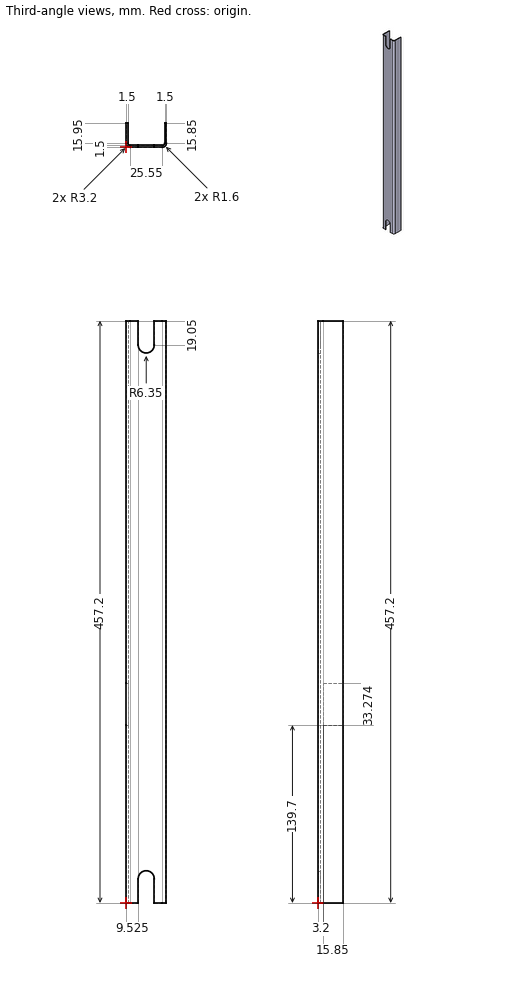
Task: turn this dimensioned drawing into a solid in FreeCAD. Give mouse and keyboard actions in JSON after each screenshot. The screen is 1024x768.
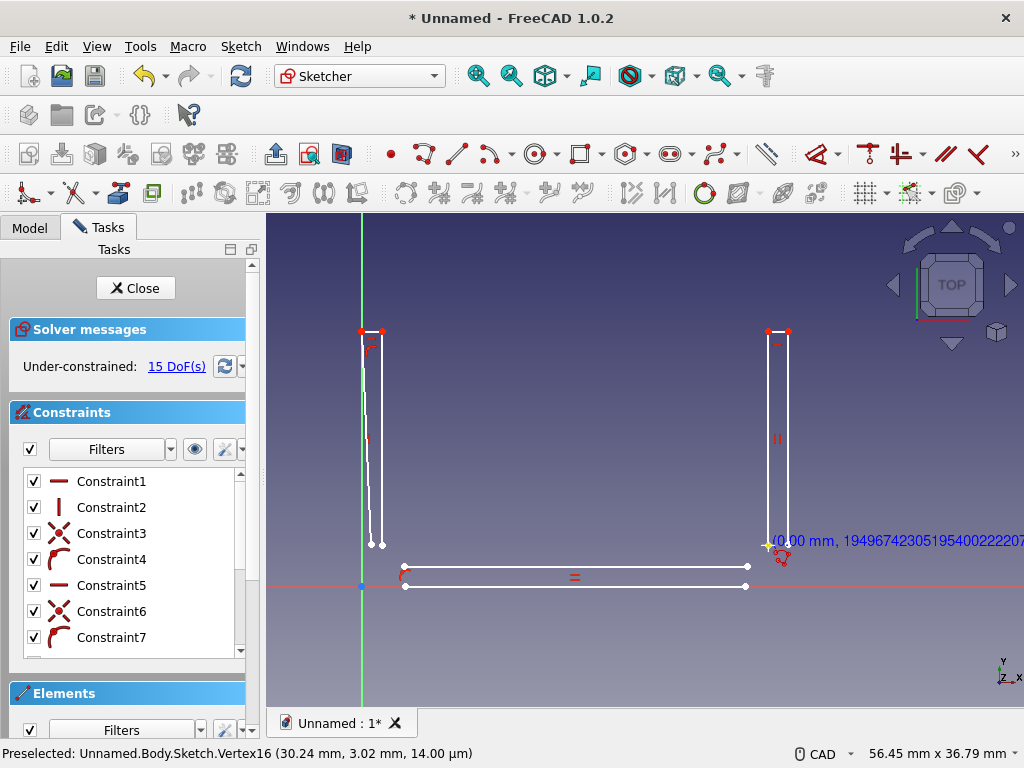
{"action": "key", "text": "g 3 a"}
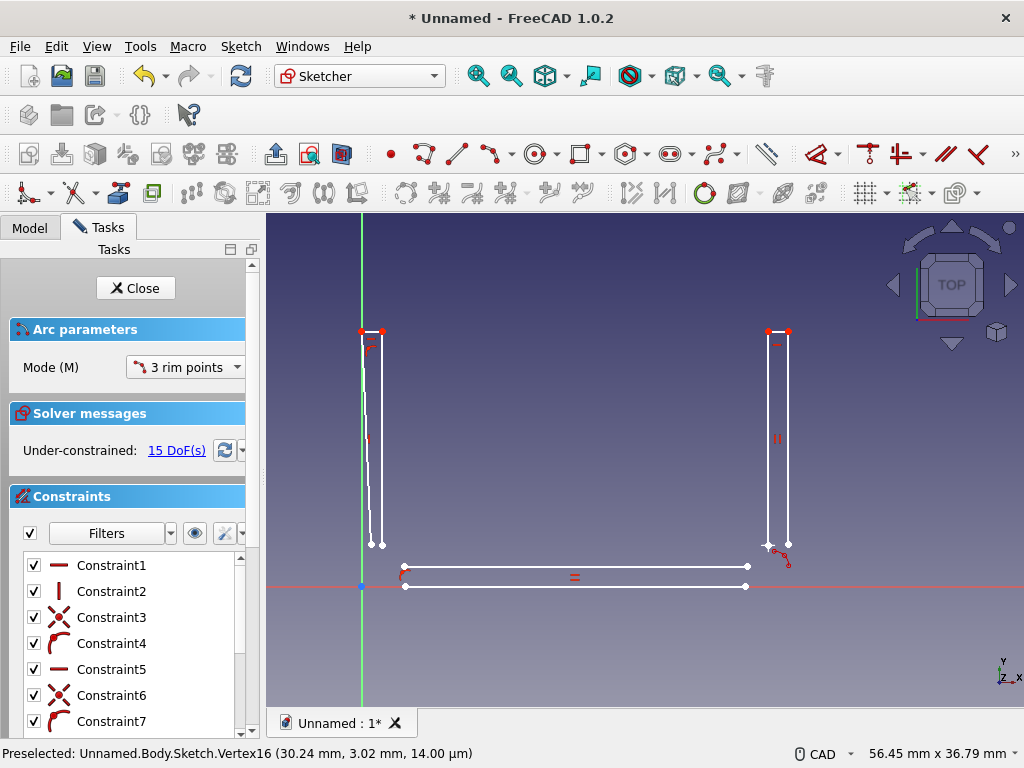
{"action": "left_click", "coordinate": [404, 567]}
{"action": "left_click", "coordinate": [382, 546]}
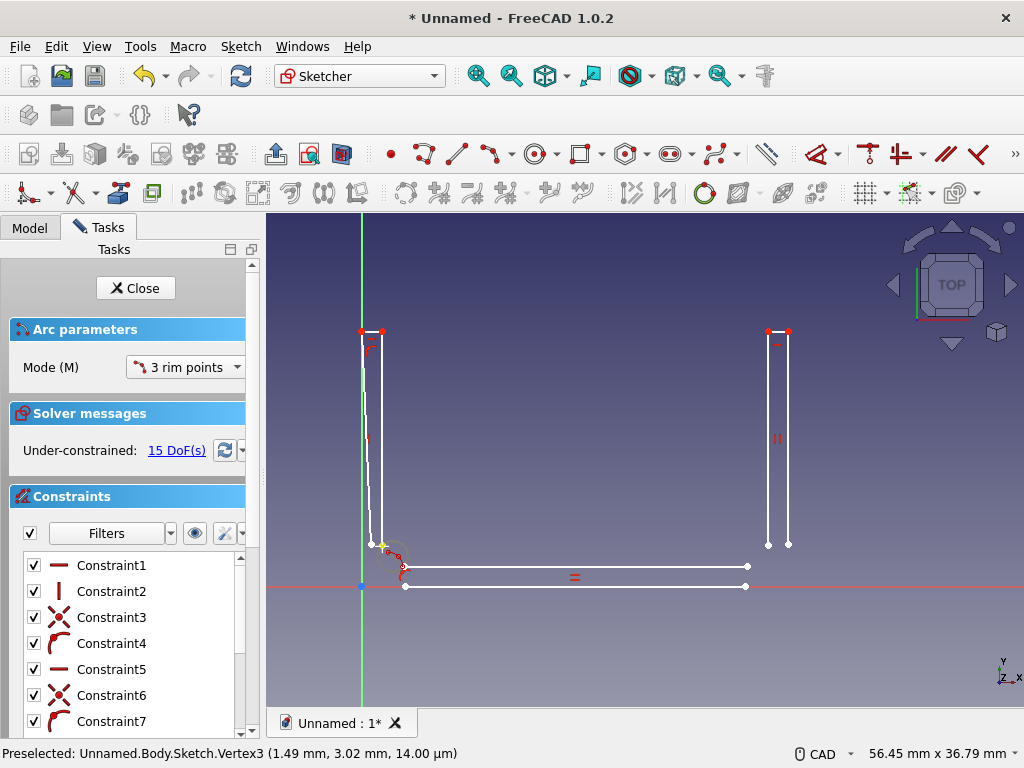
{"action": "scroll", "coordinate": [388, 560], "scroll_direction": "up", "scroll_amount": 5}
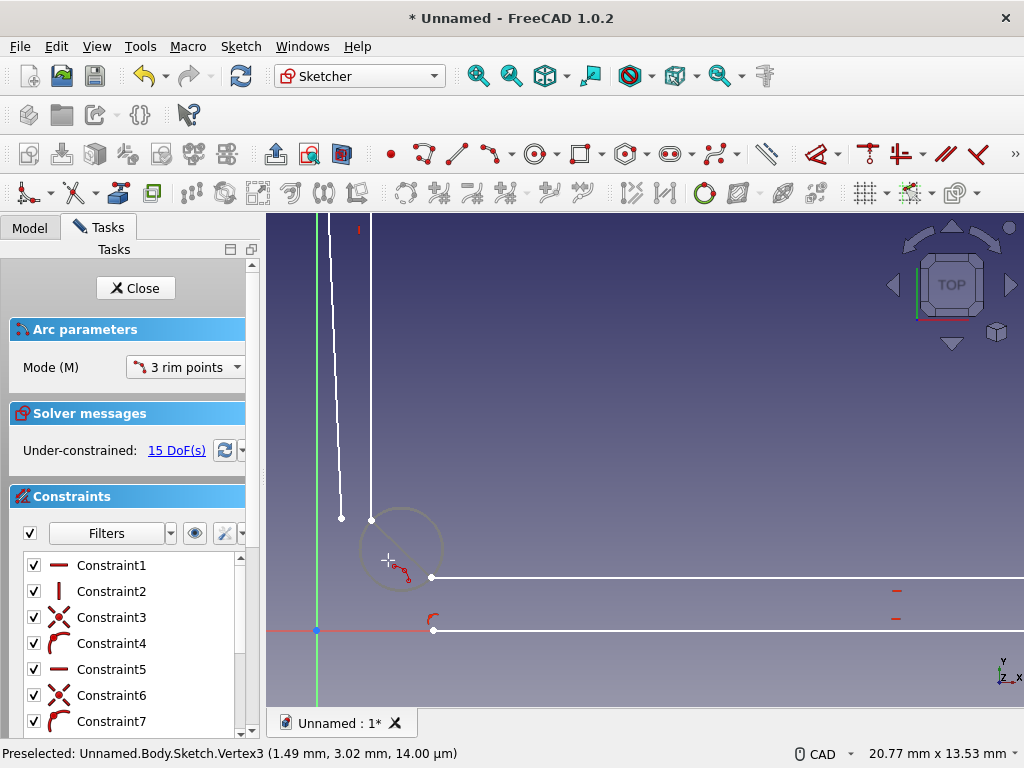
{"action": "left_click", "coordinate": [389, 559]}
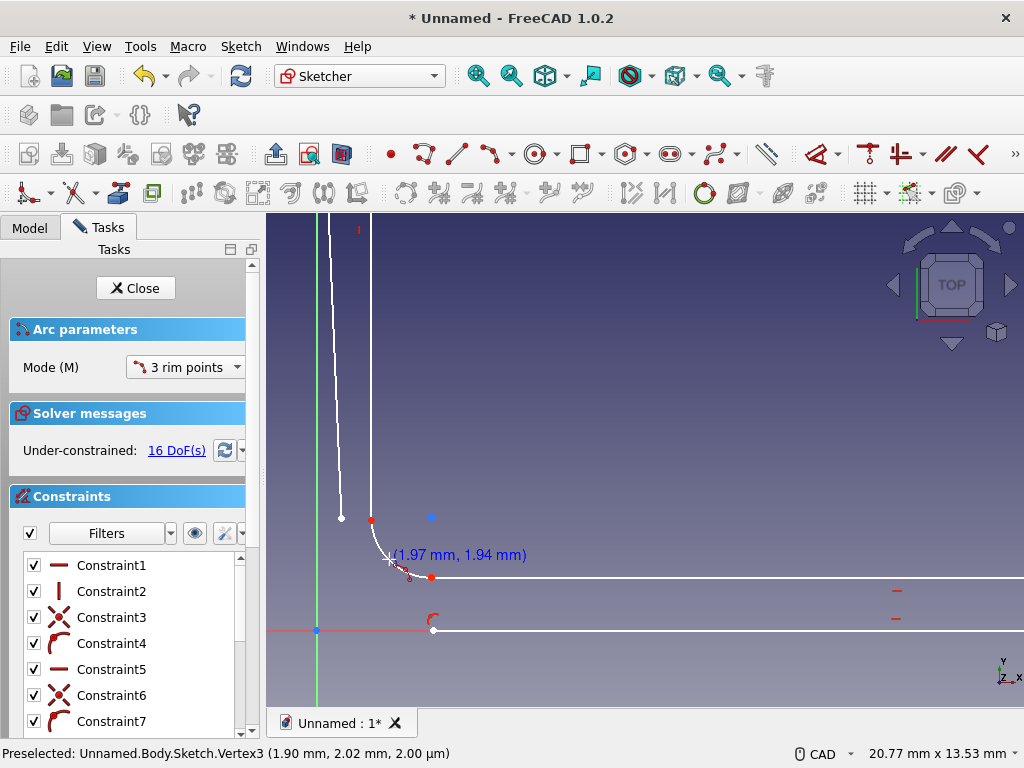
{"action": "left_click", "coordinate": [342, 518]}
{"action": "left_click", "coordinate": [434, 631]}
{"action": "left_click", "coordinate": [351, 597]}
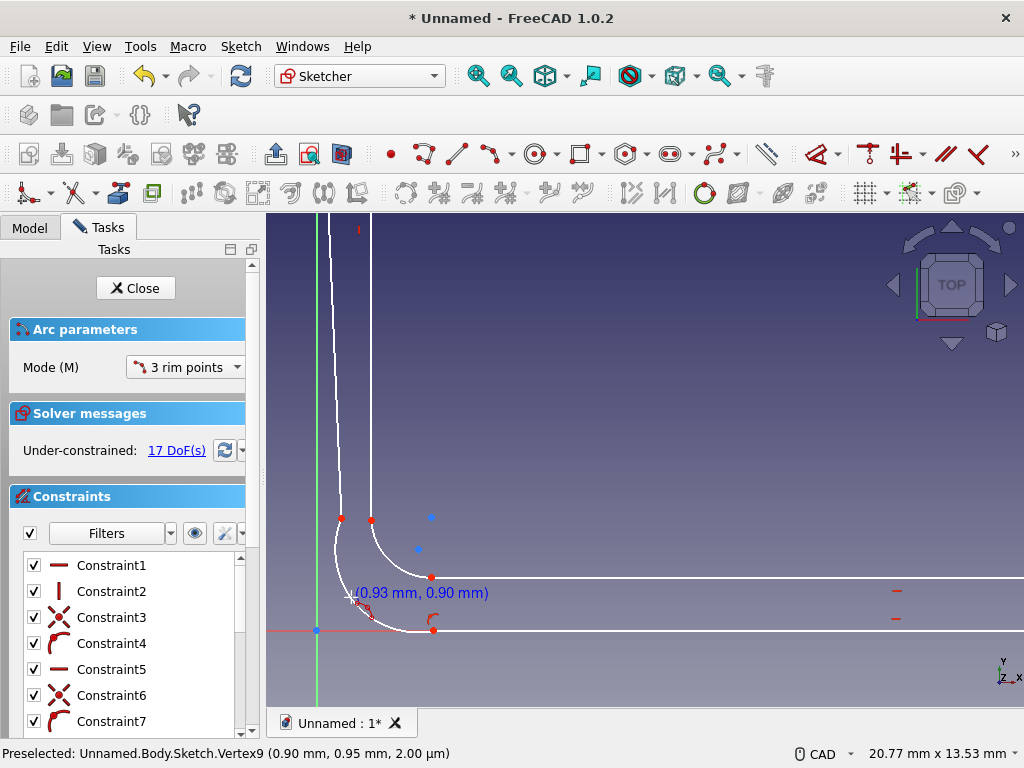
{"action": "scroll", "coordinate": [390, 563], "scroll_direction": "down", "scroll_amount": 5}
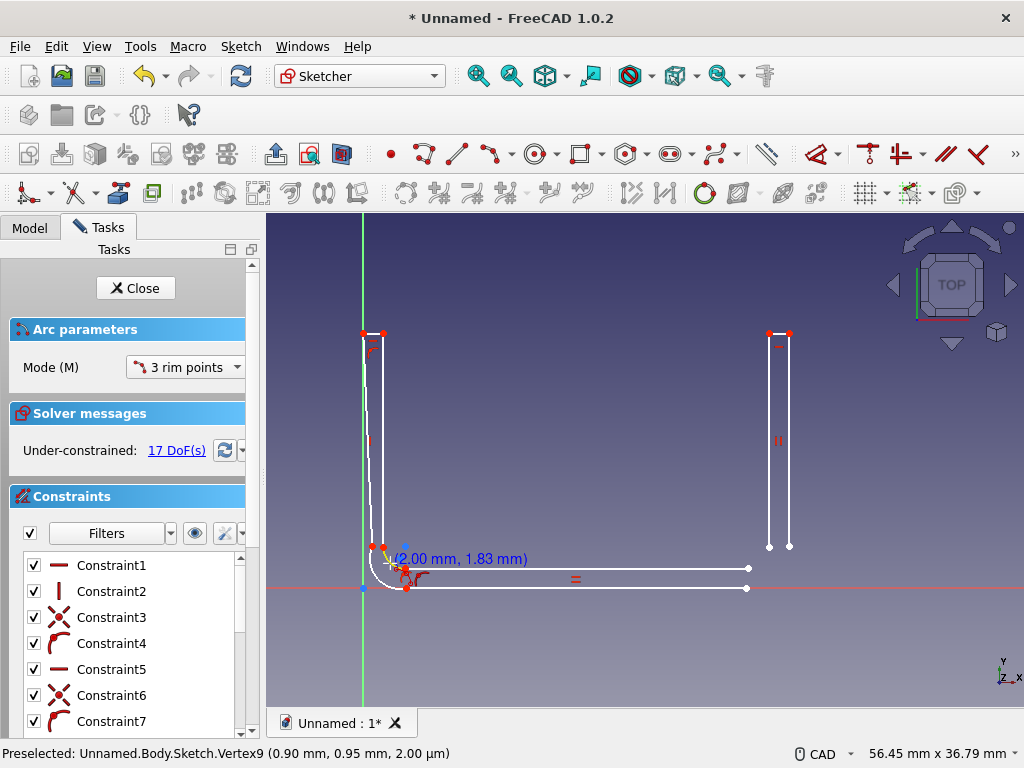
{"action": "left_click", "coordinate": [746, 588]}
{"action": "left_click", "coordinate": [789, 547]}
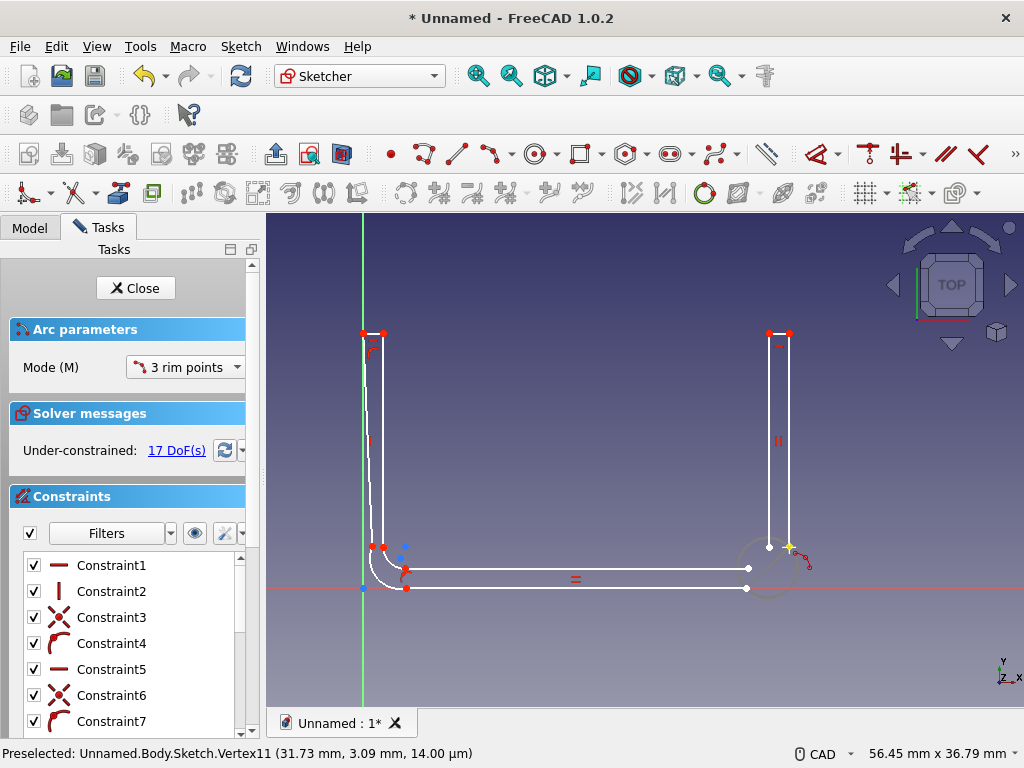
{"action": "scroll", "coordinate": [777, 576], "scroll_direction": "up", "scroll_amount": 2}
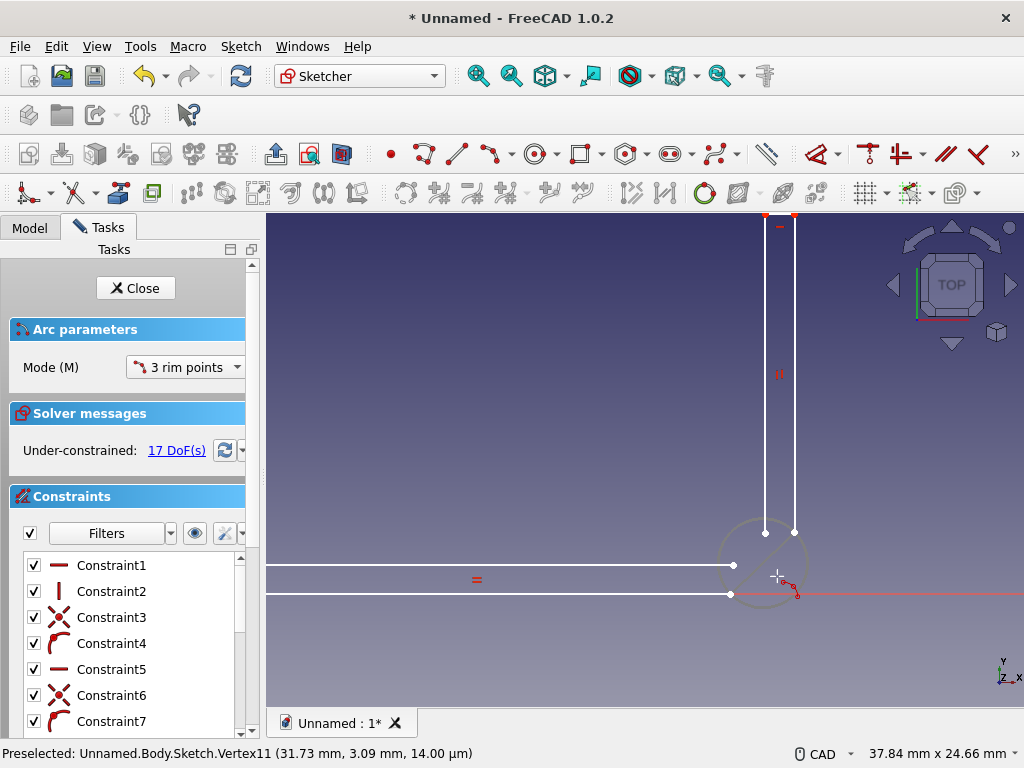
{"action": "left_click", "coordinate": [777, 575]}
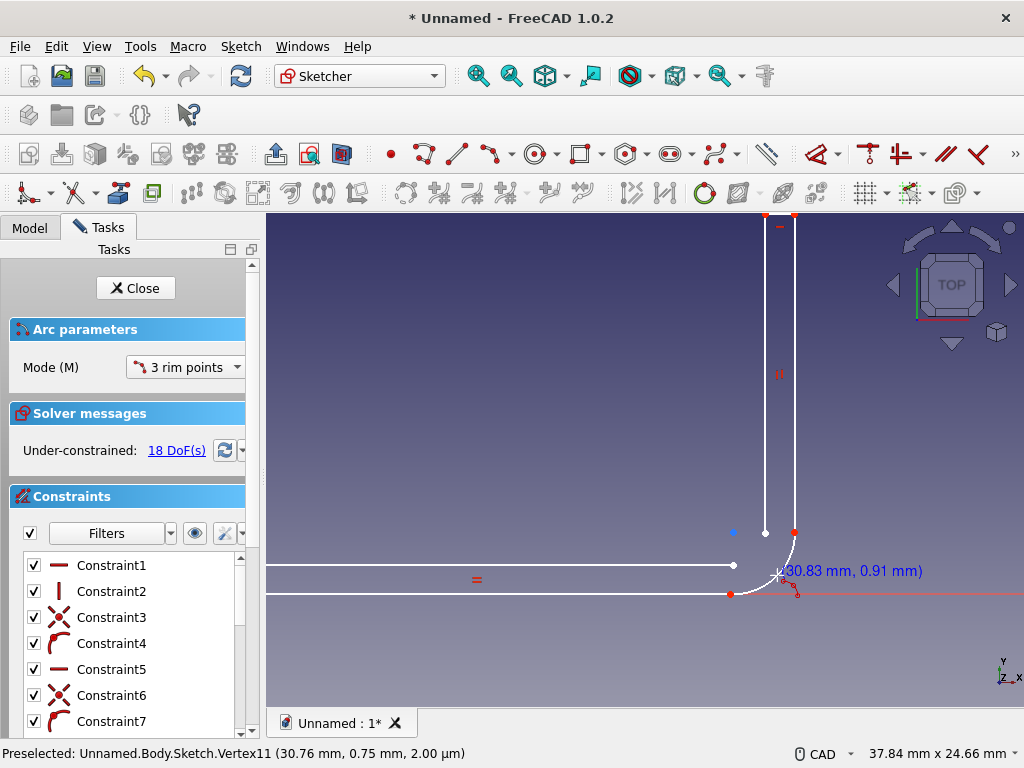
{"action": "left_click", "coordinate": [765, 534]}
{"action": "left_click", "coordinate": [734, 565]}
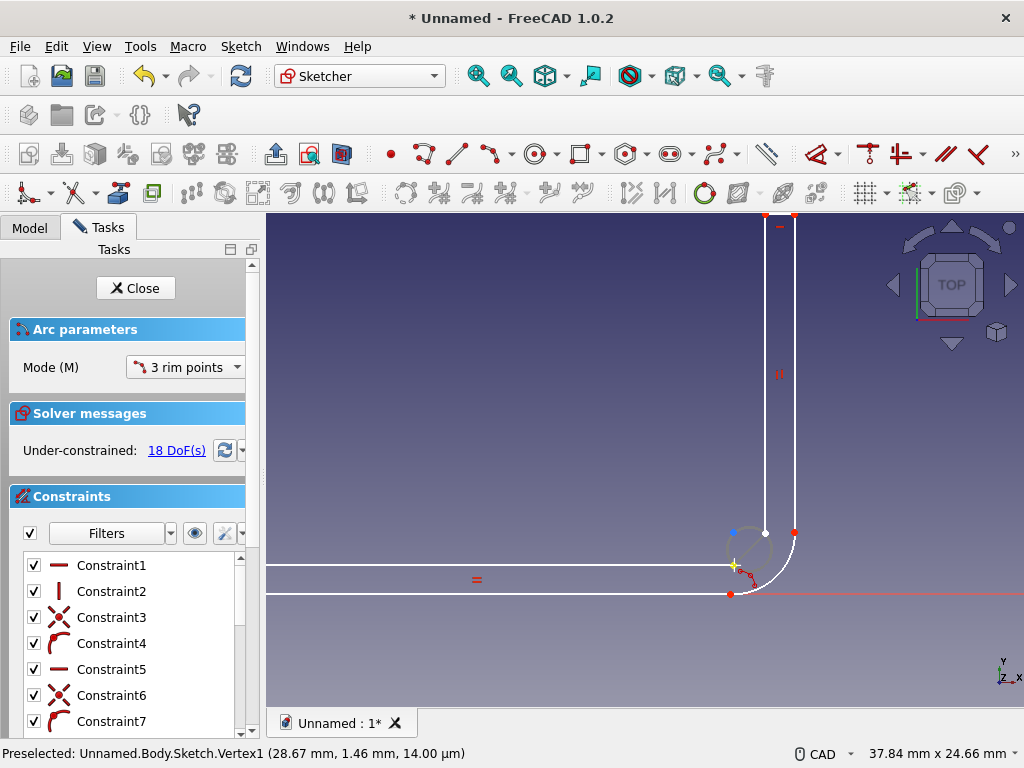
{"action": "scroll", "coordinate": [756, 555], "scroll_direction": "up", "scroll_amount": 3}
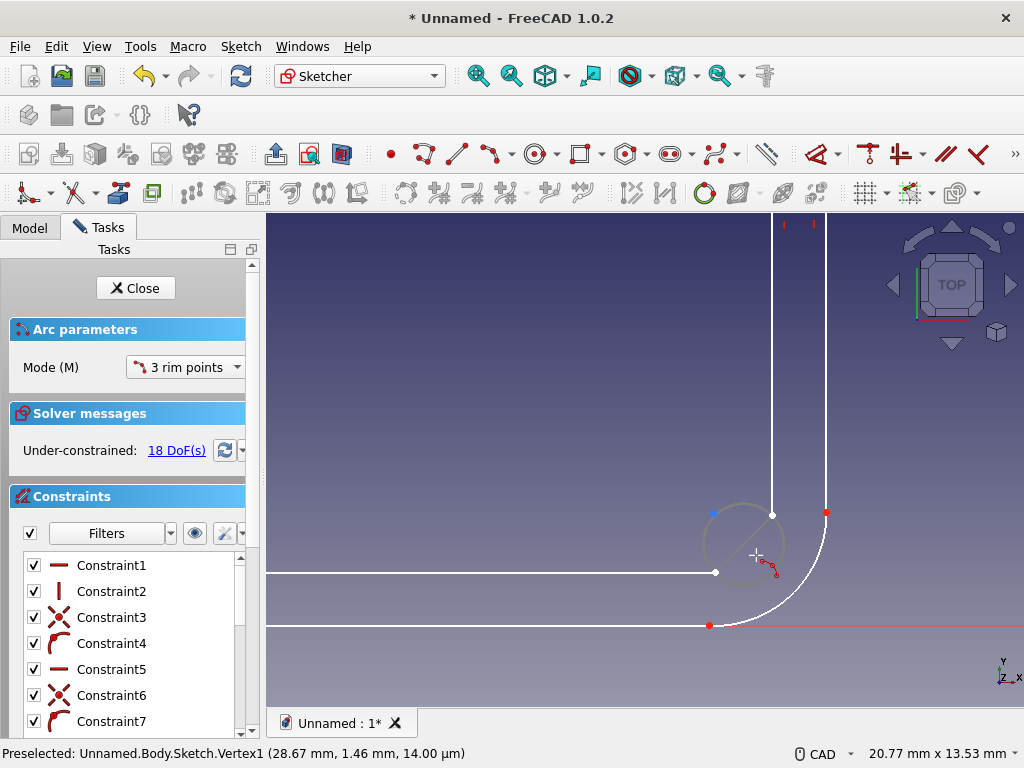
{"action": "left_click", "coordinate": [755, 554]}
{"action": "key", "text": "Escape"}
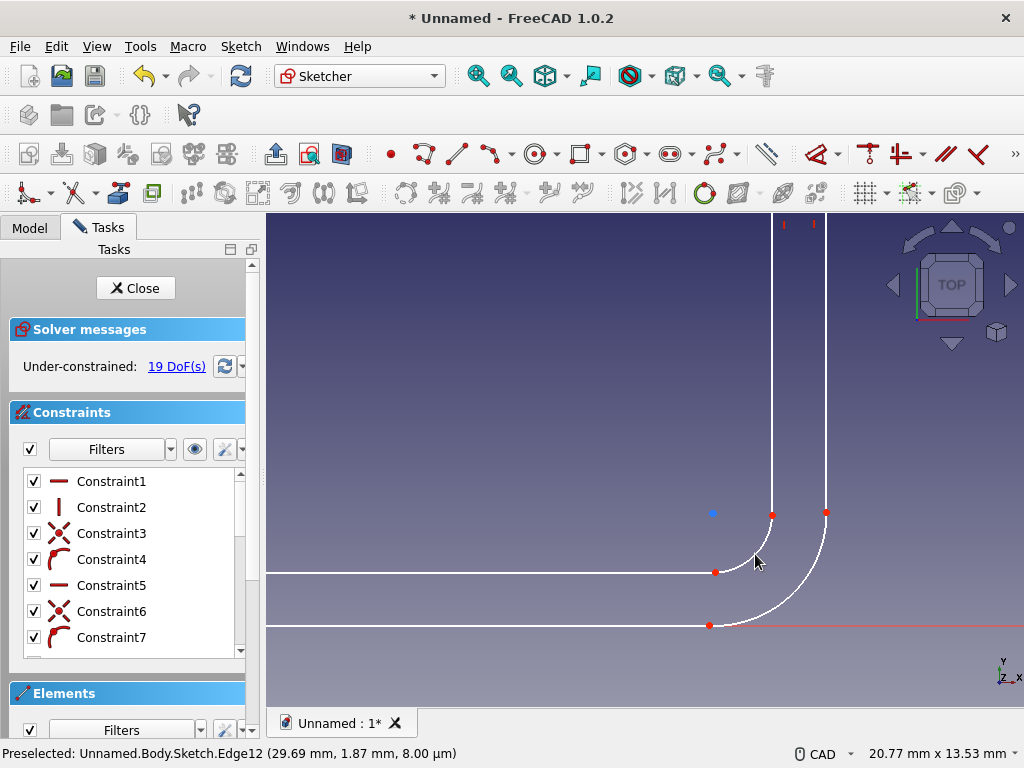
{"action": "left_click", "coordinate": [435, 573]}